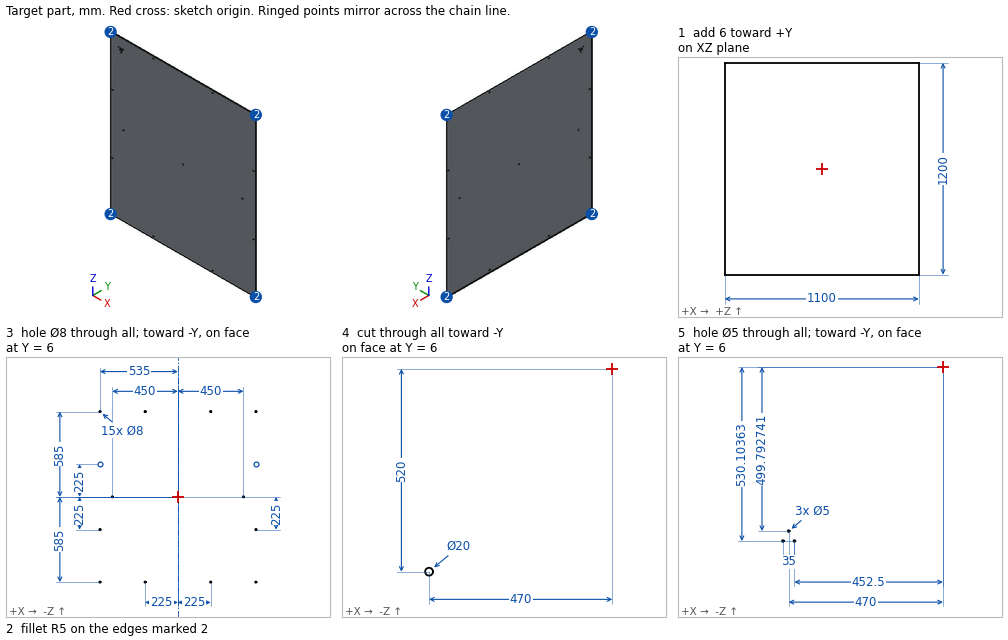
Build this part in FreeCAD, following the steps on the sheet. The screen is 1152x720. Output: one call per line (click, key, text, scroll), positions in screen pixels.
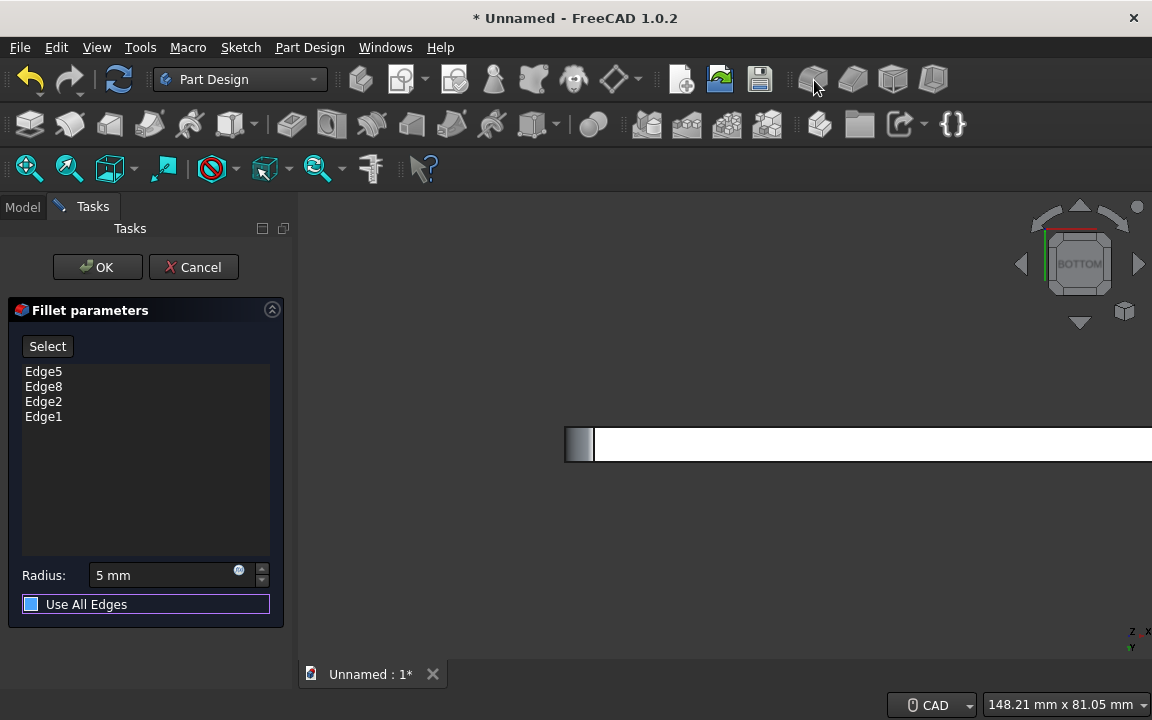
click(98, 267)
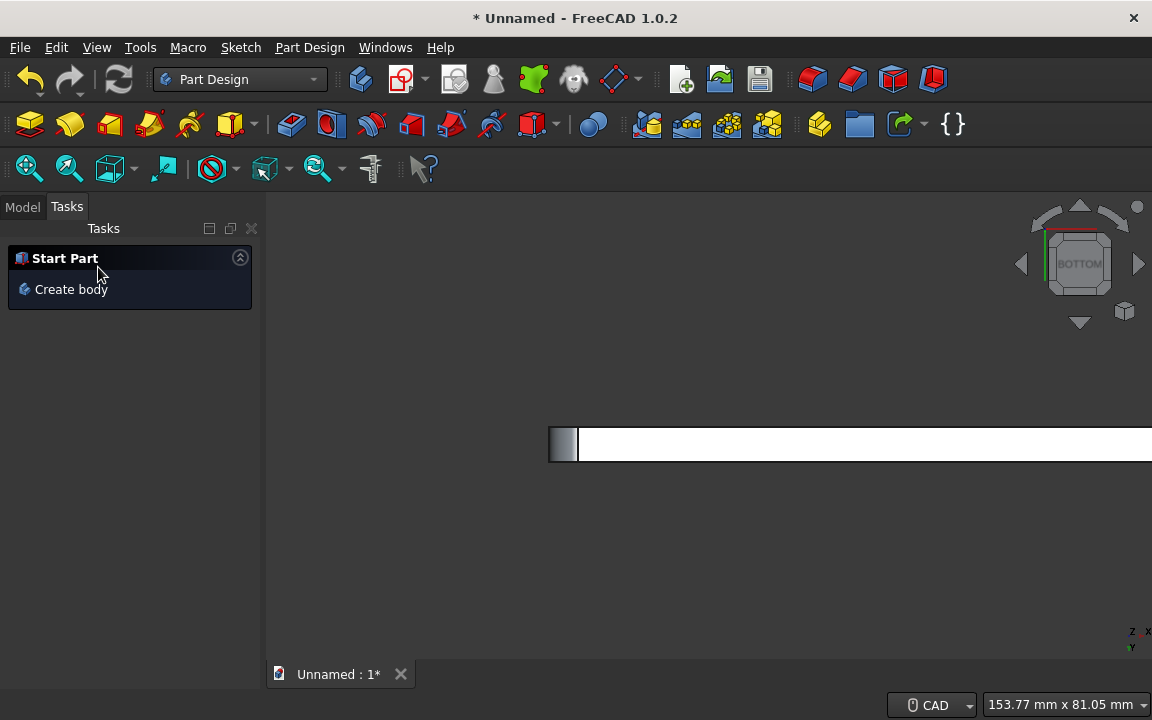
click(30, 170)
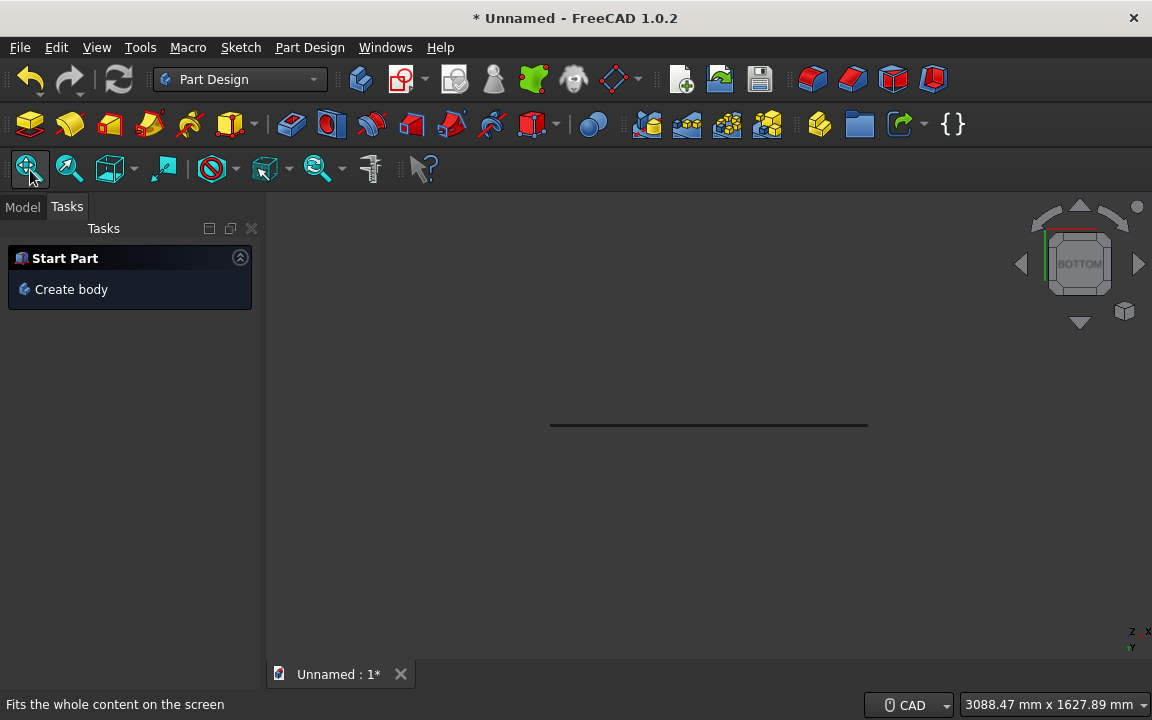
key(4)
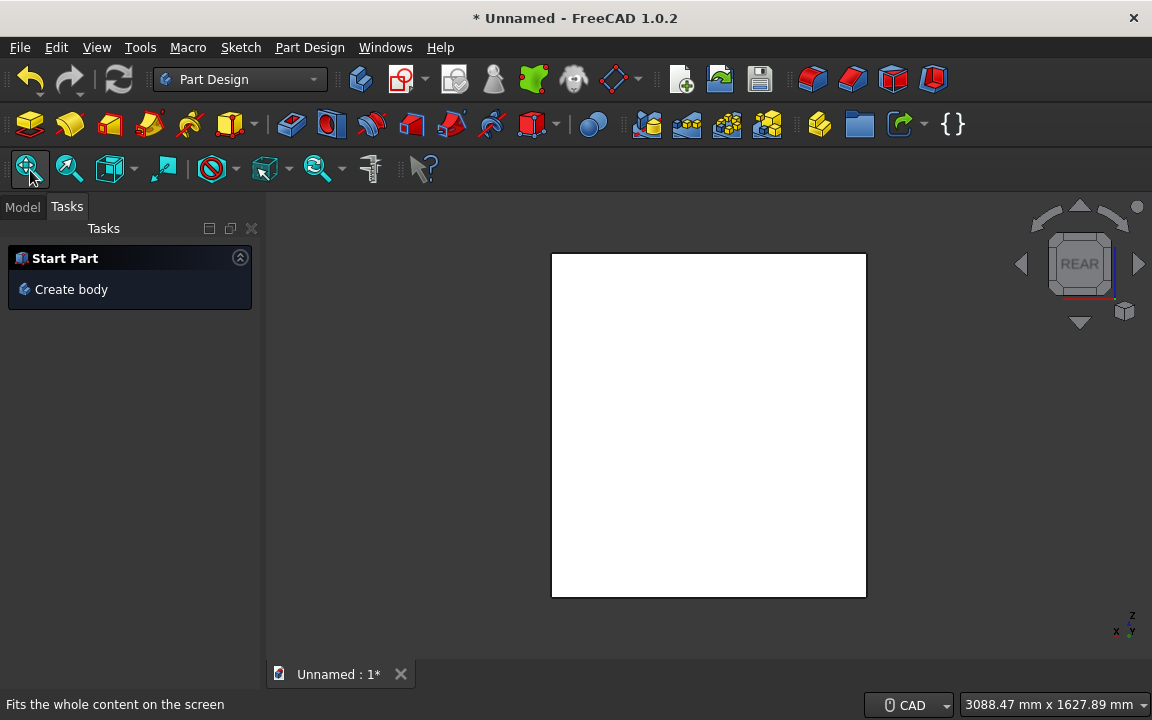
click(709, 425)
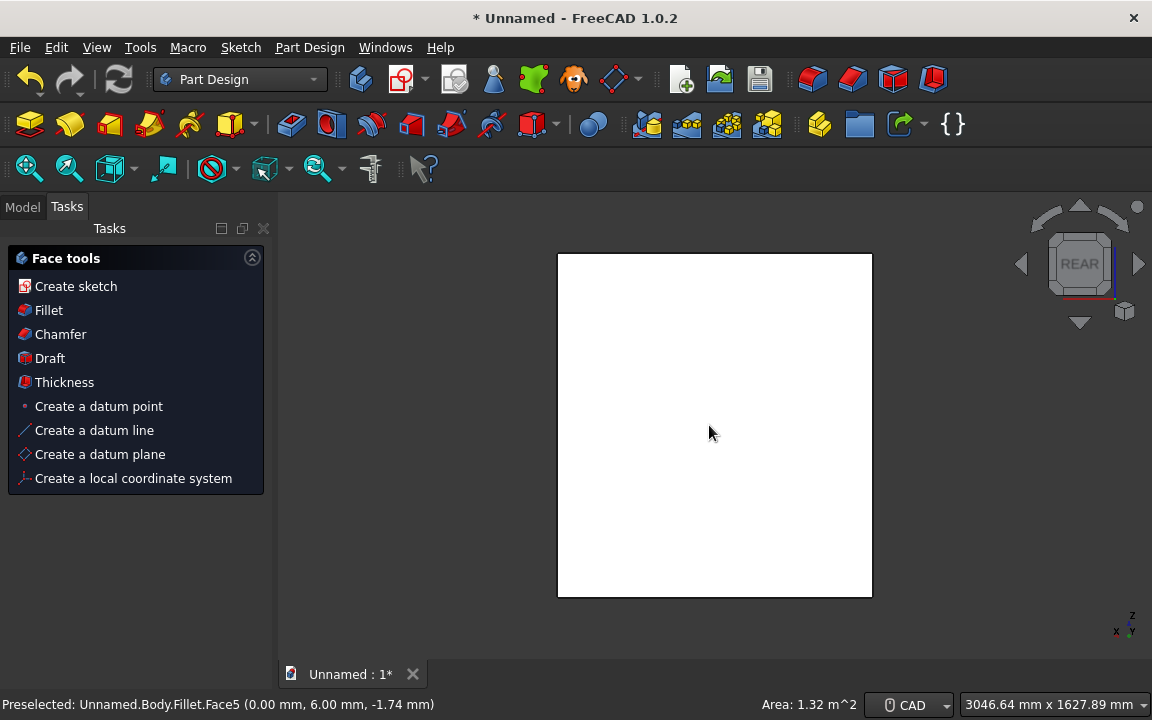
click(402, 80)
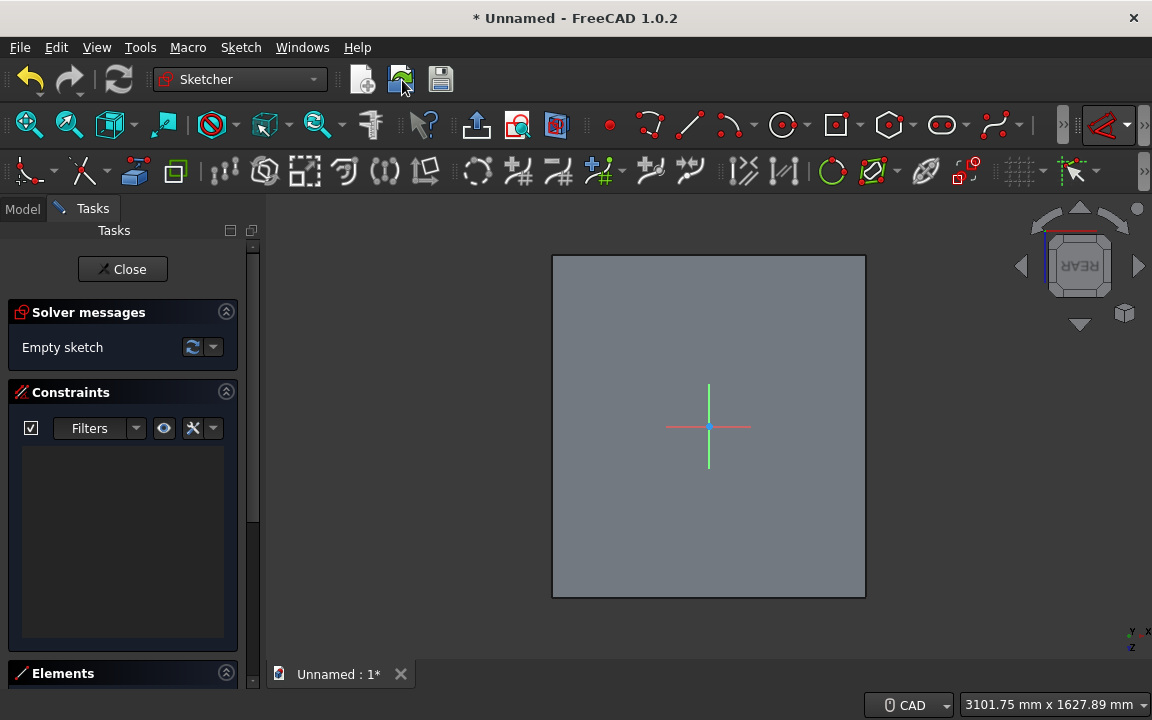
click(784, 126)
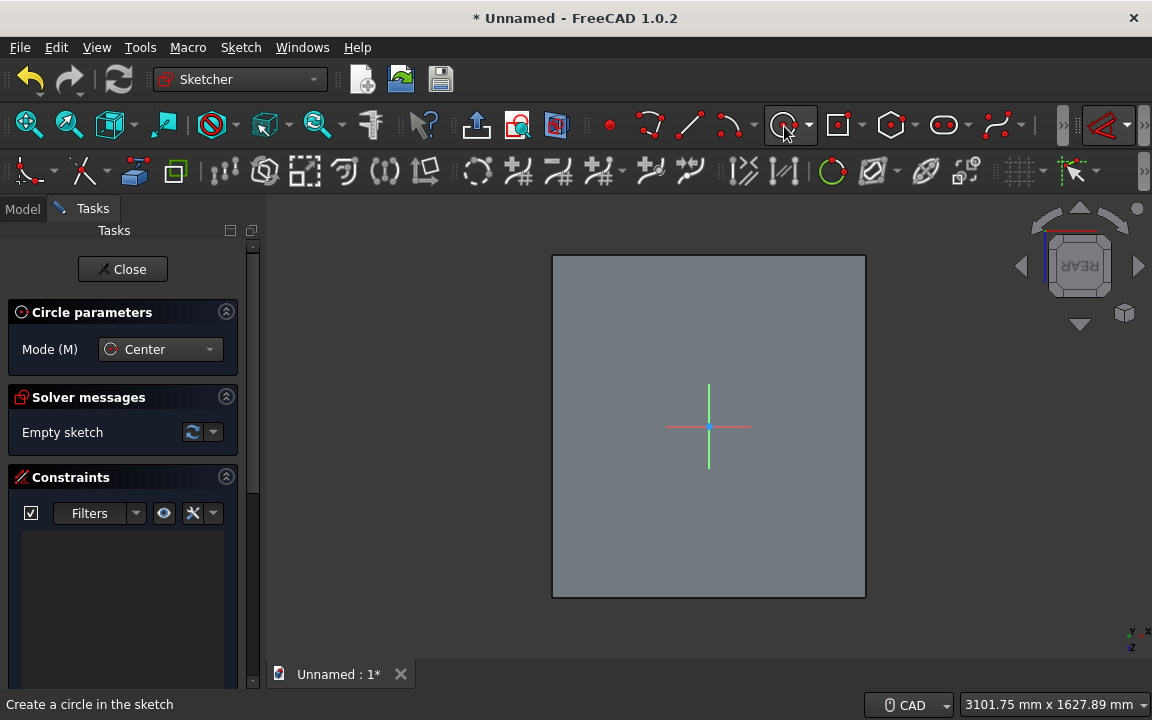
scroll(556, 259, up, 15)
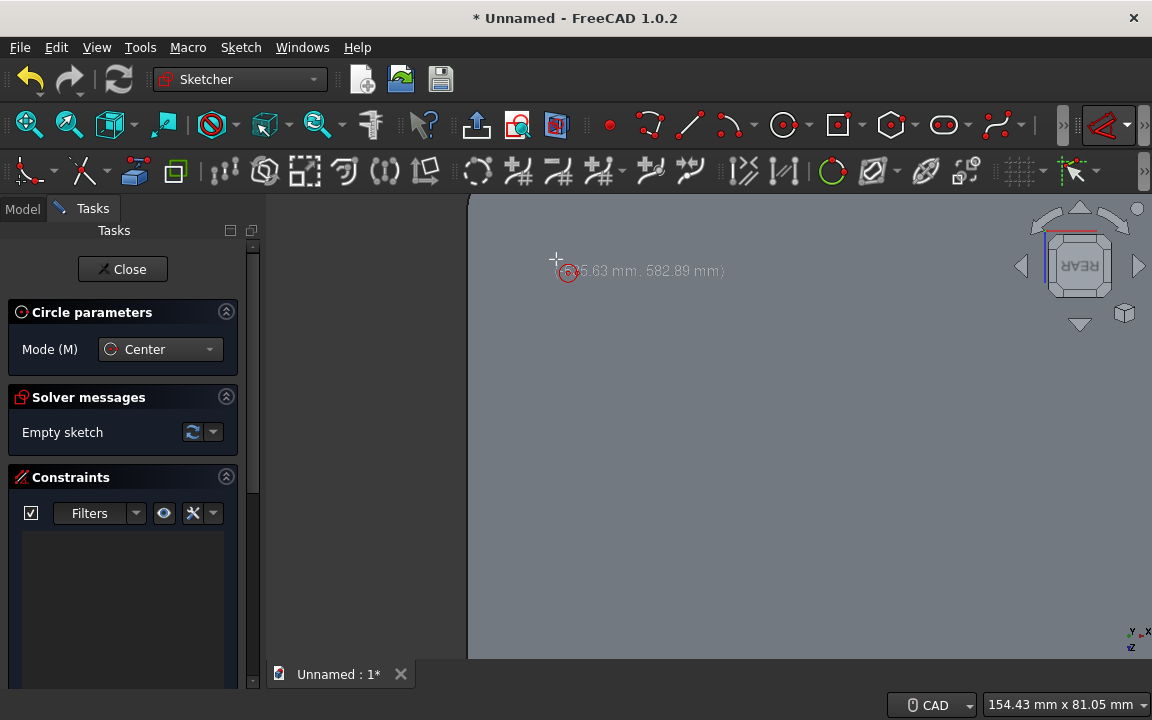
scroll(484, 259, down, 15)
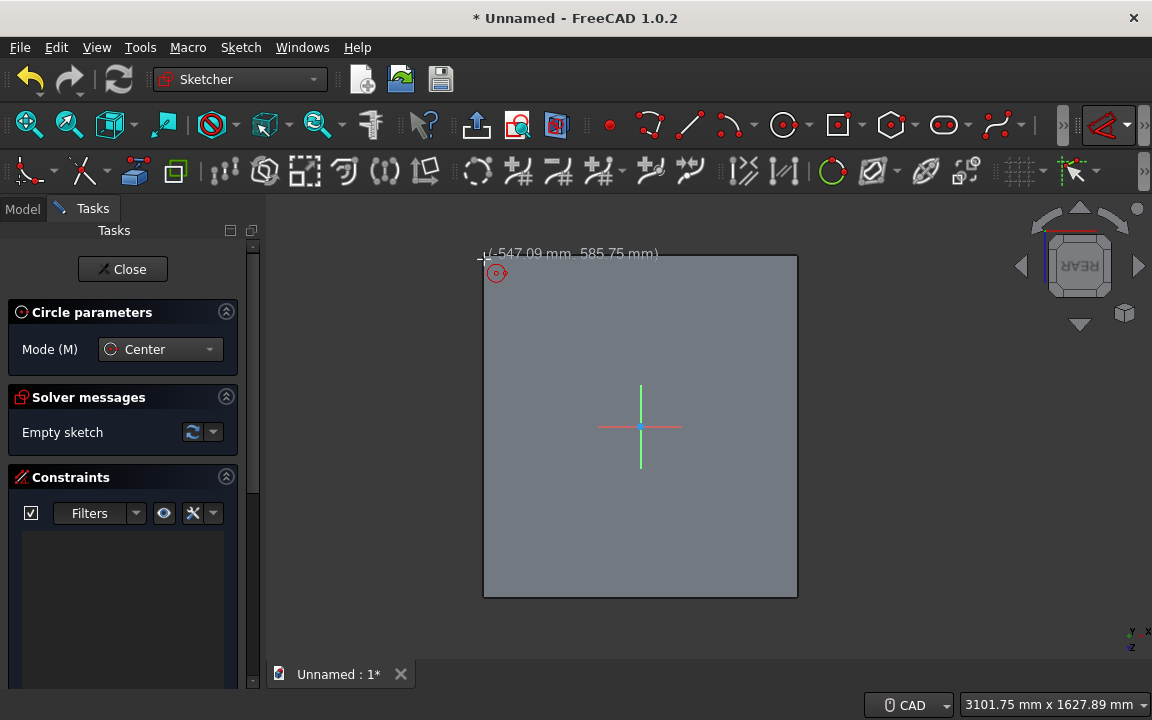
click(488, 259)
move(488, 259)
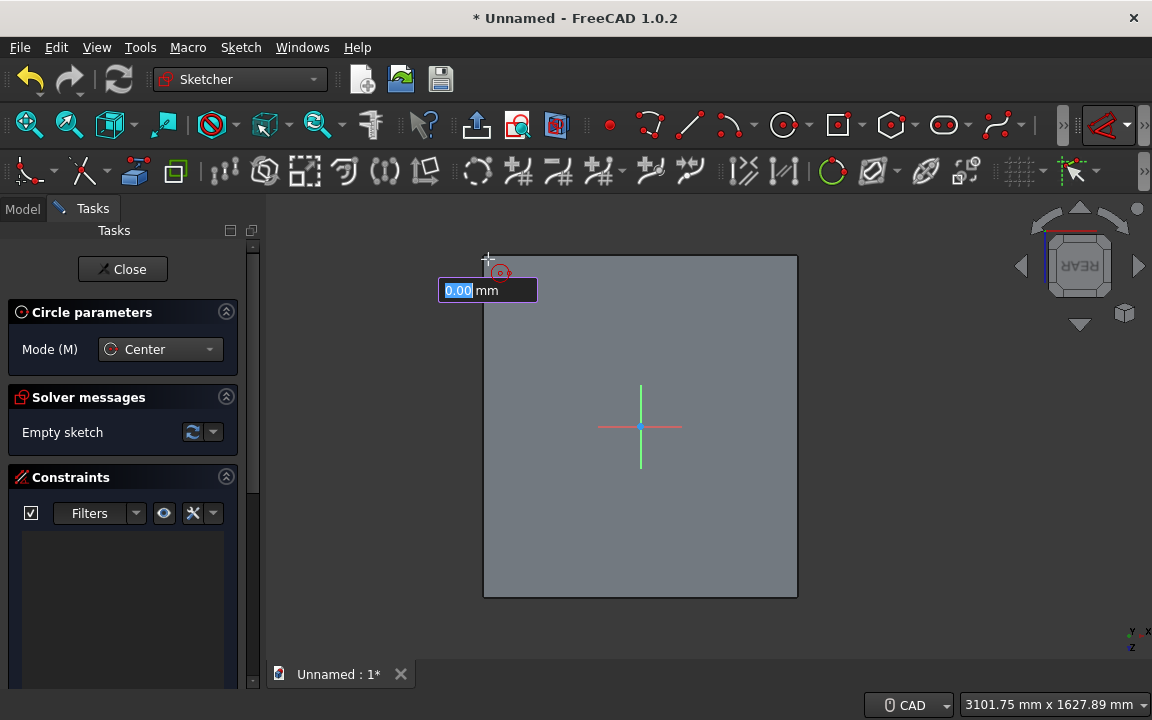
text(8)
key(Return)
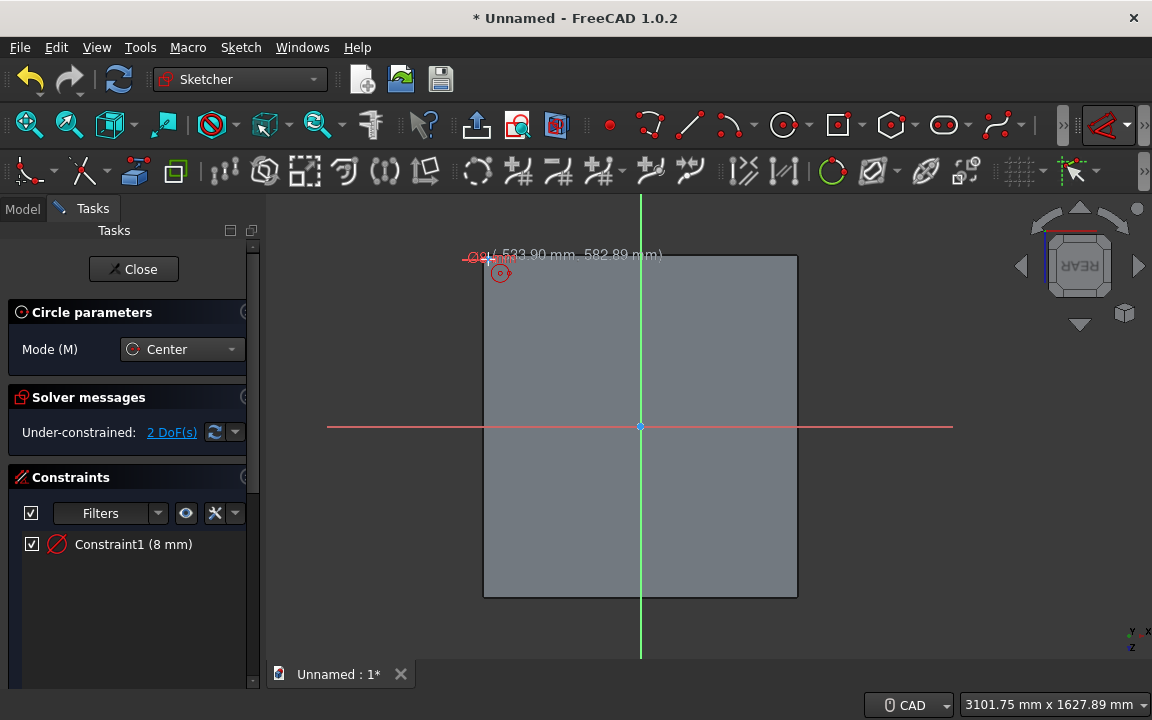
scroll(793, 259, up, 15)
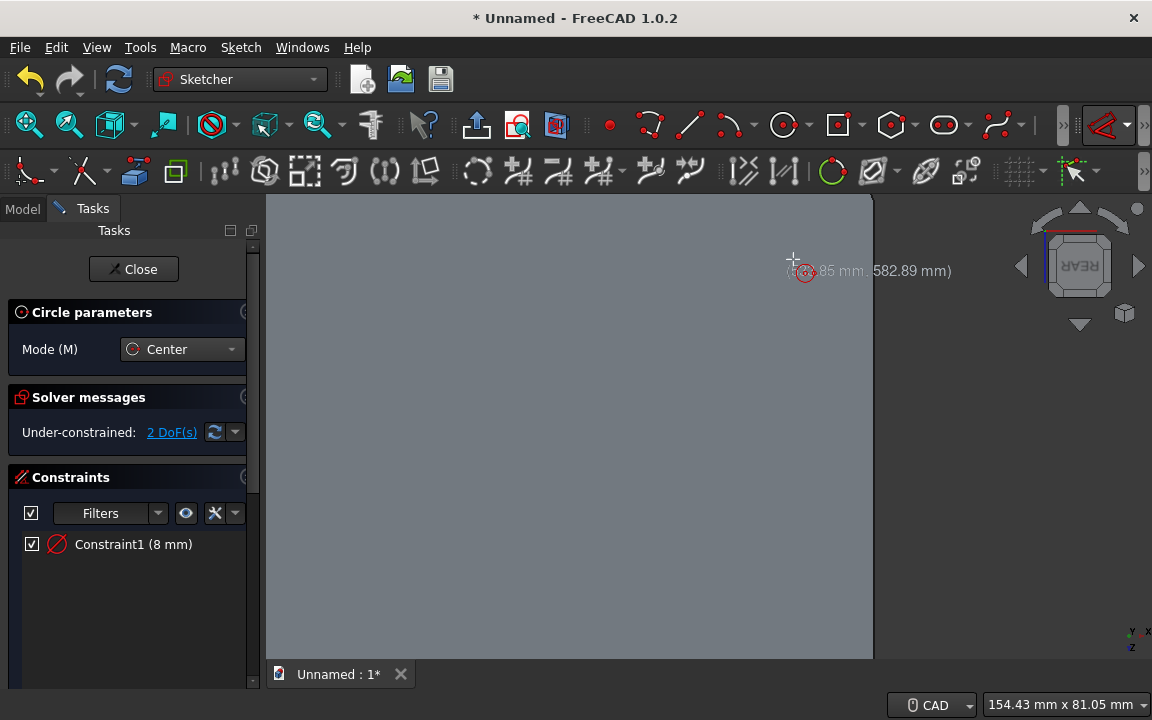
scroll(794, 259, down, 15)